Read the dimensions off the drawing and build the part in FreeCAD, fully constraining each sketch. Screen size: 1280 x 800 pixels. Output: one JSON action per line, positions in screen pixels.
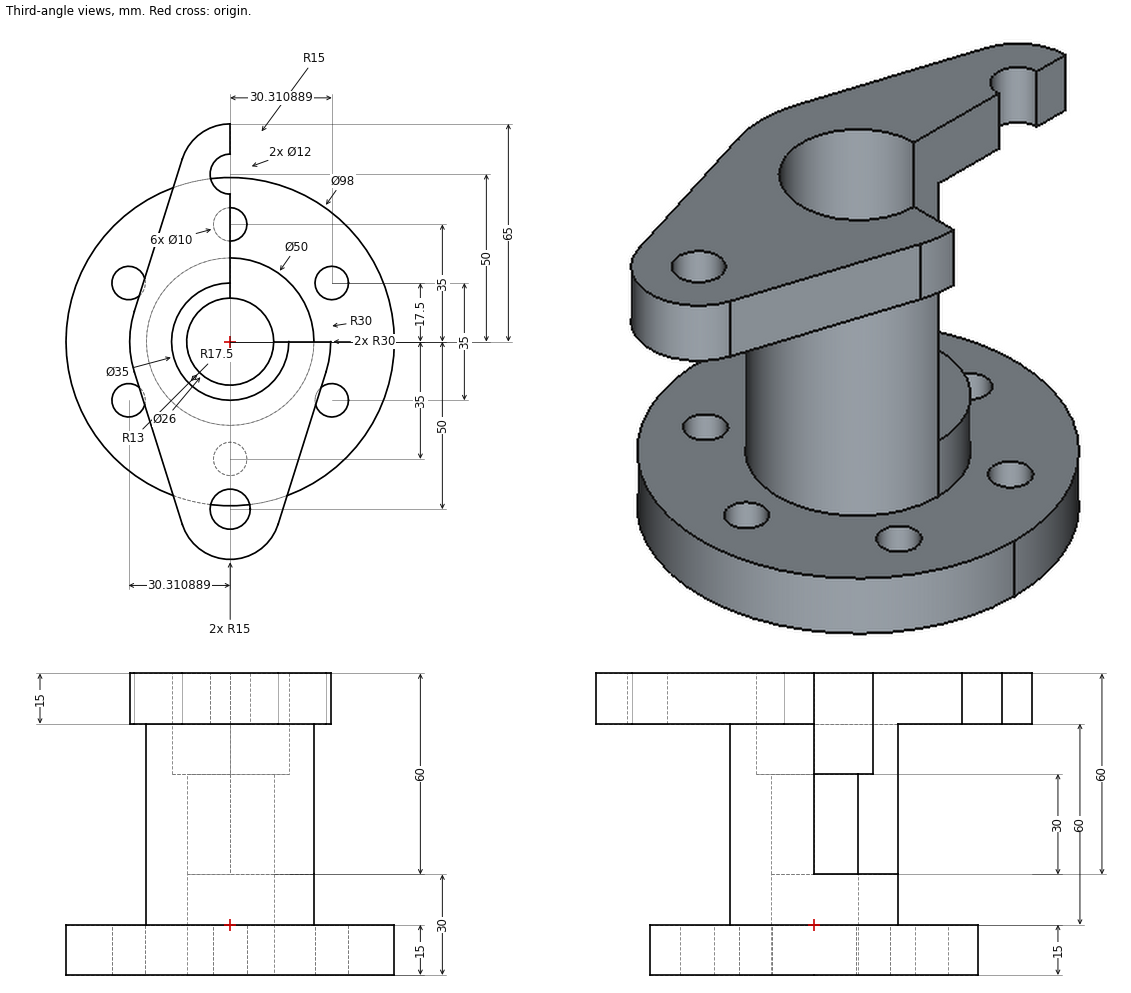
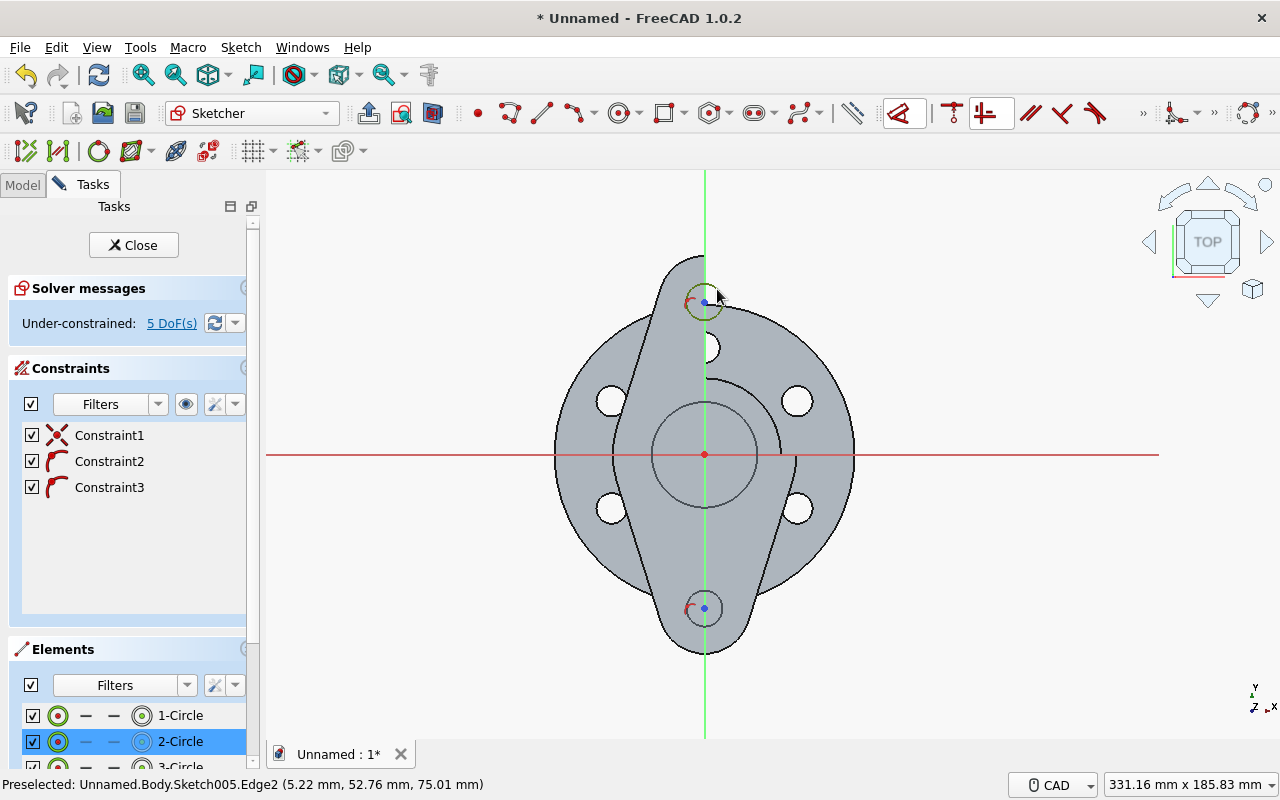
{"action": "left_click", "coordinate": [717, 596]}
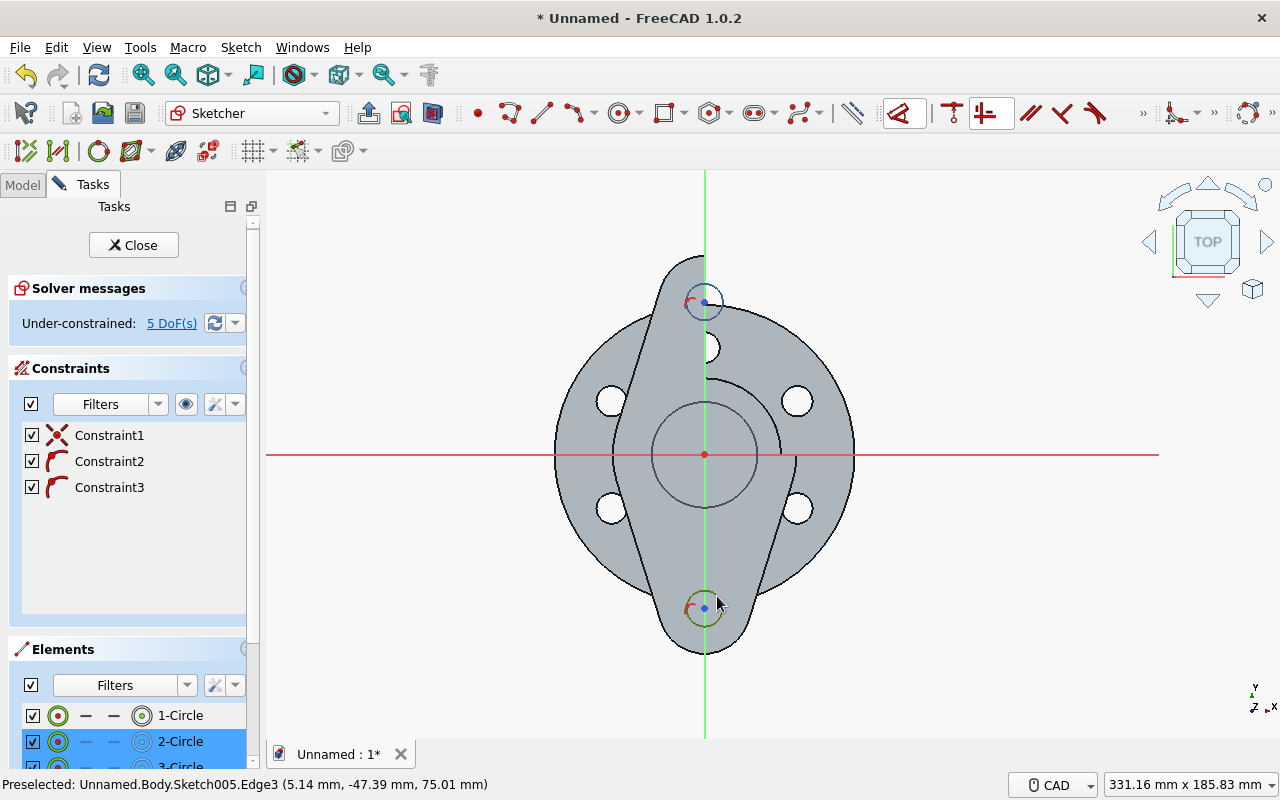
{"action": "key", "text": "e"}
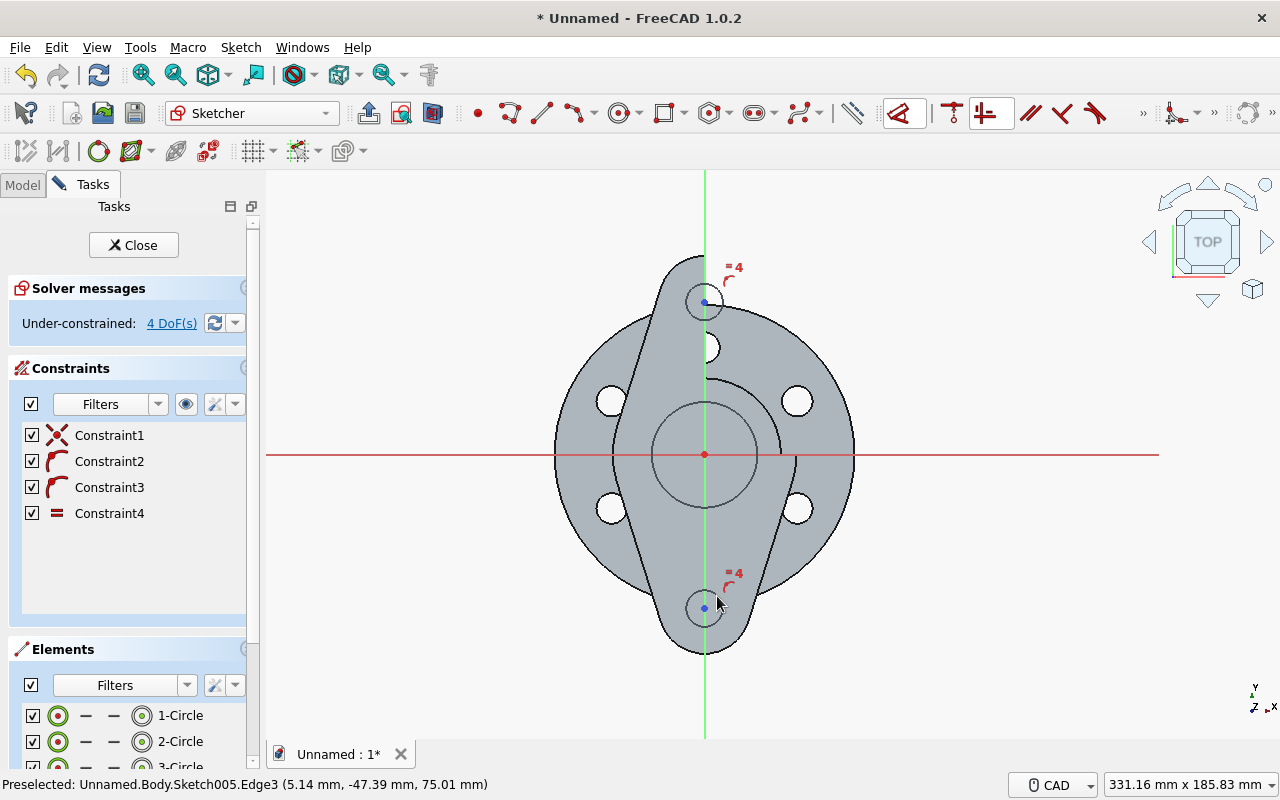
{"action": "left_click", "coordinate": [742, 417]}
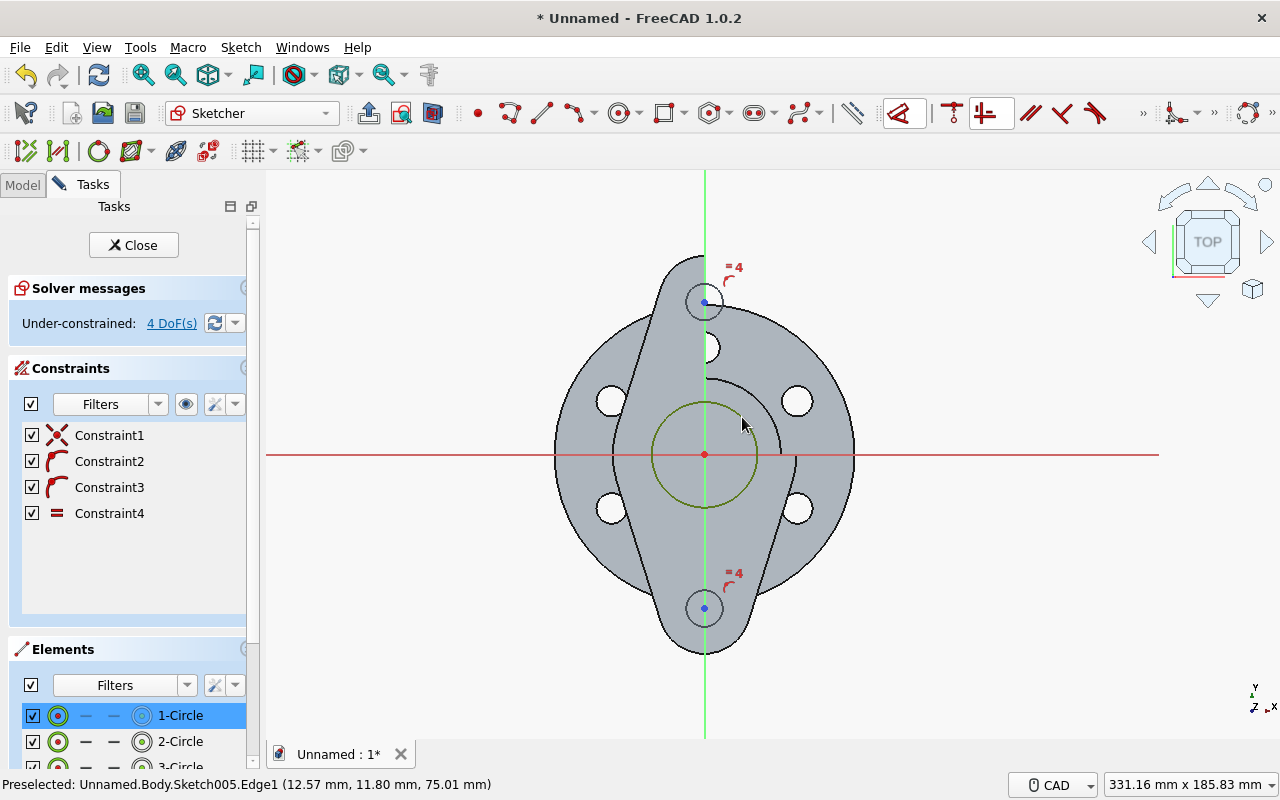
{"action": "key", "text": "k o"}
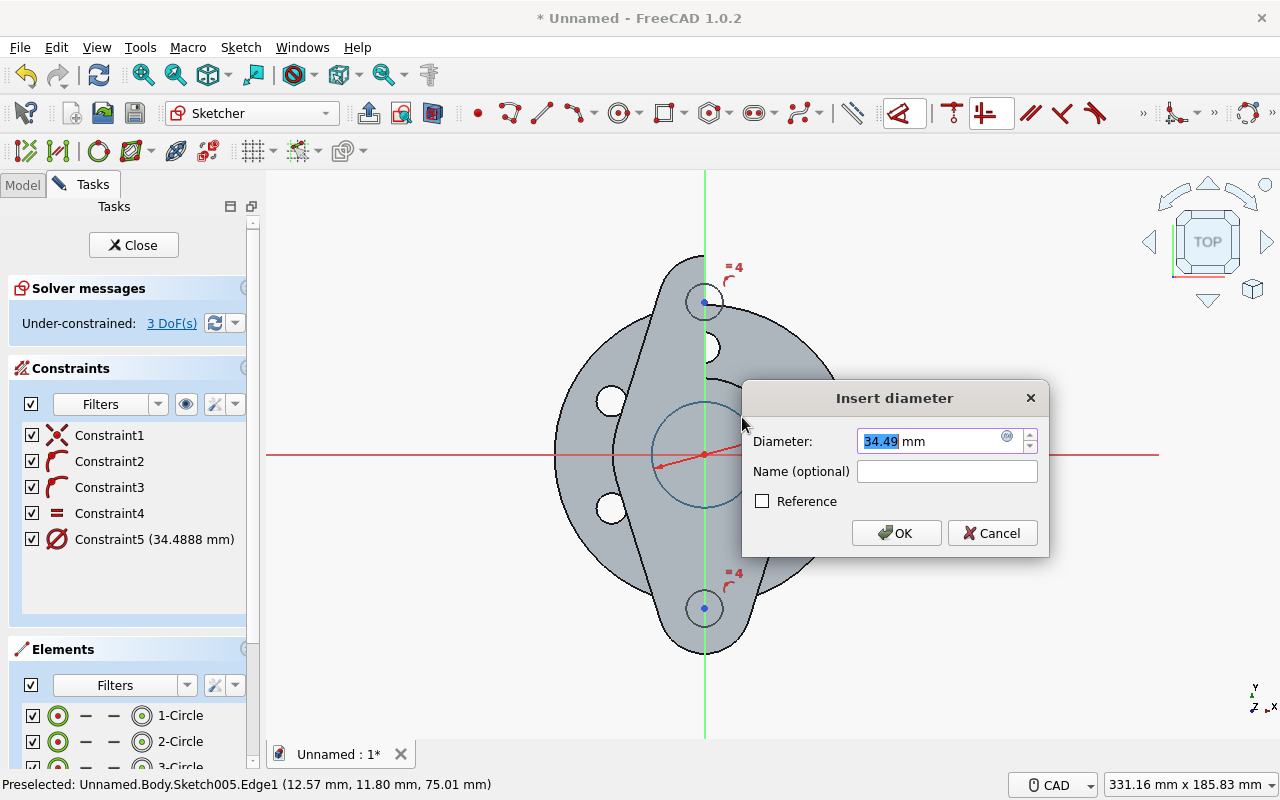
{"action": "type", "text": "35"}
{"action": "key", "text": "Return"}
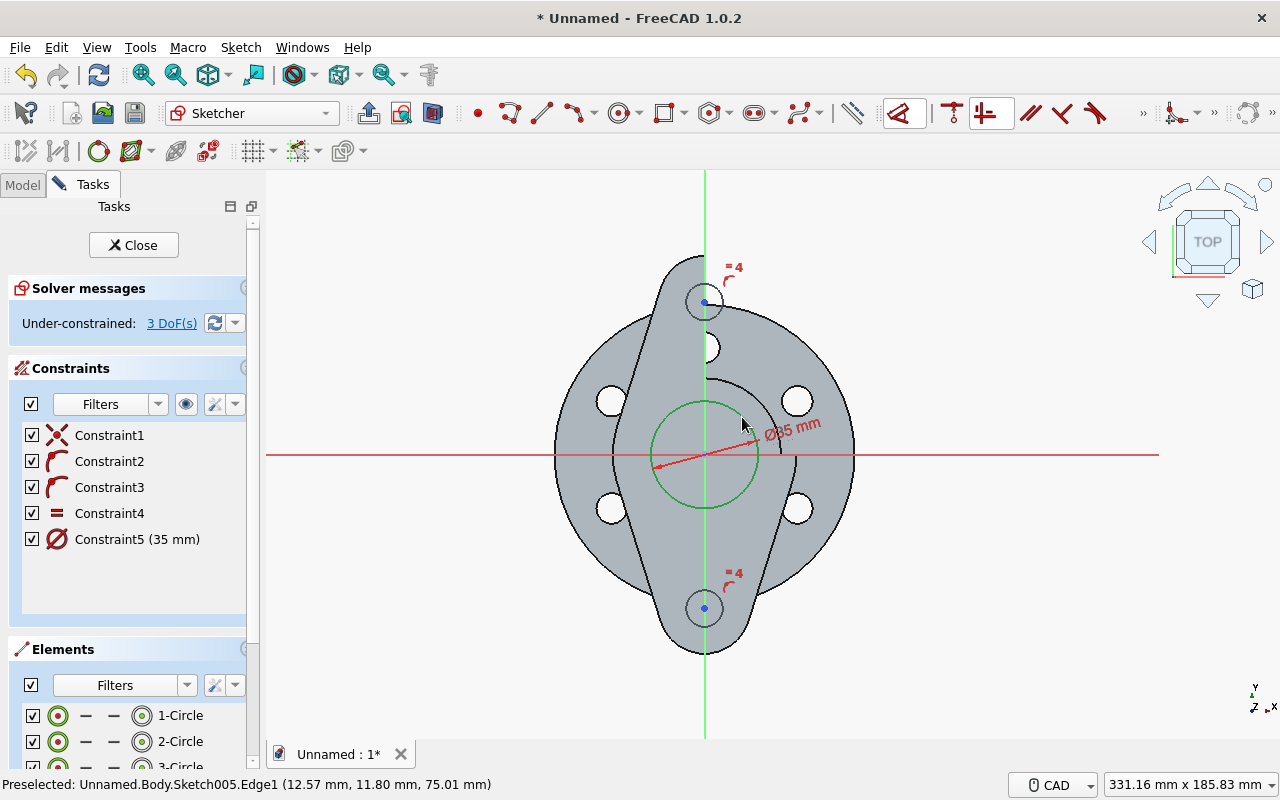
{"action": "left_click", "coordinate": [717, 289]}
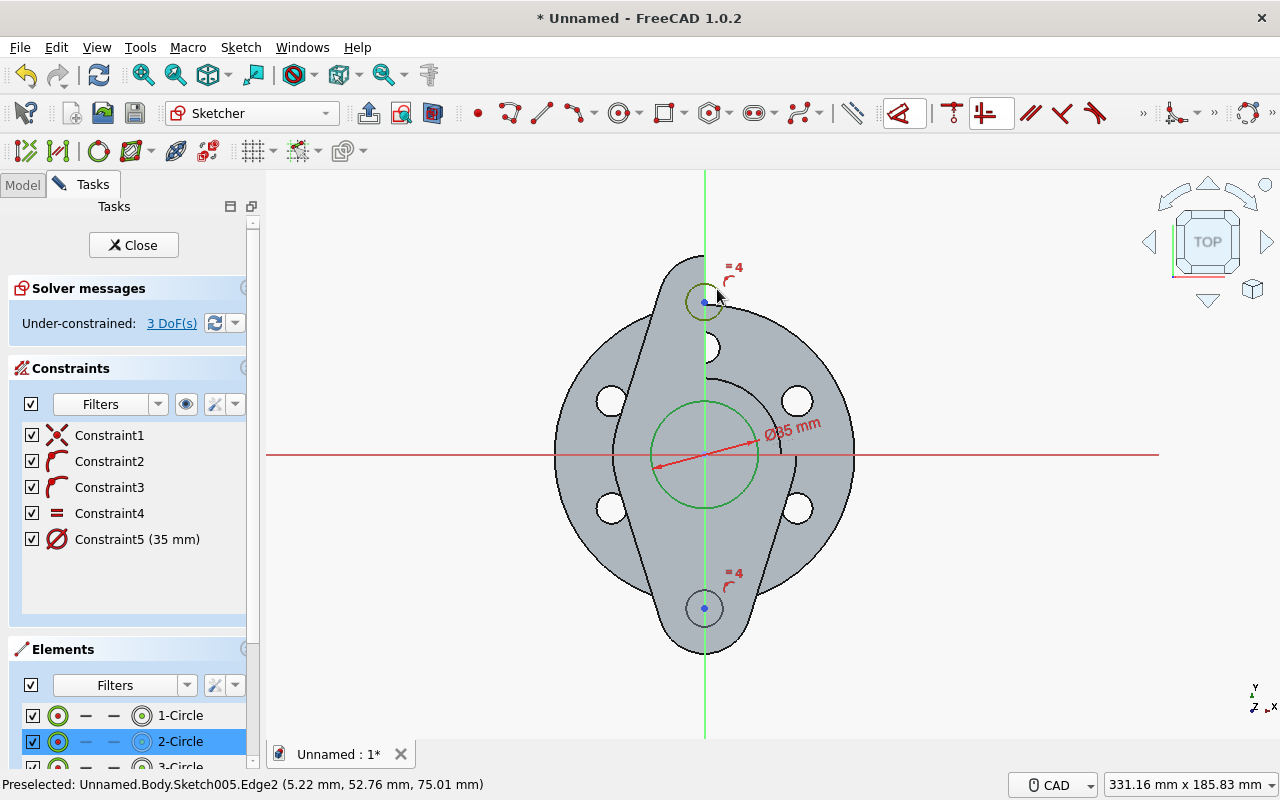
{"action": "key", "text": "k o"}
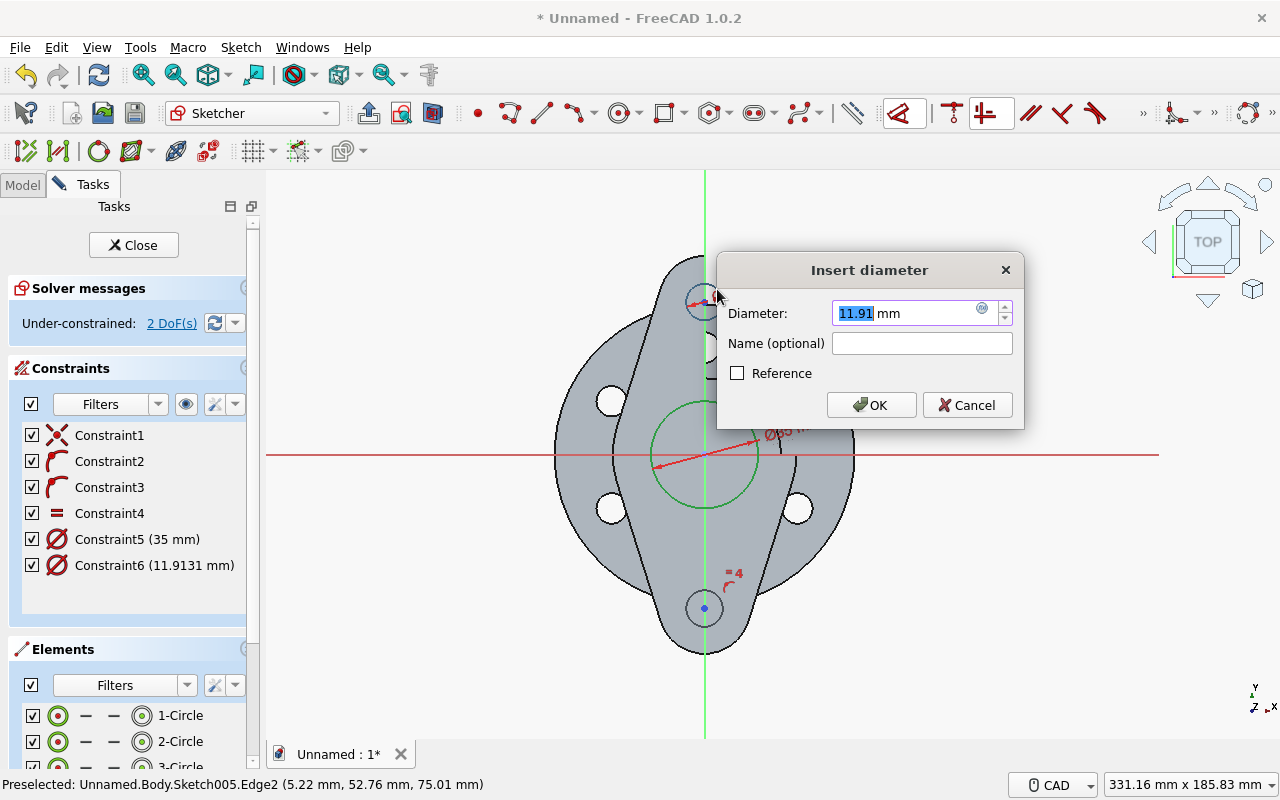
{"action": "type", "text": "12"}
{"action": "key", "text": "Return"}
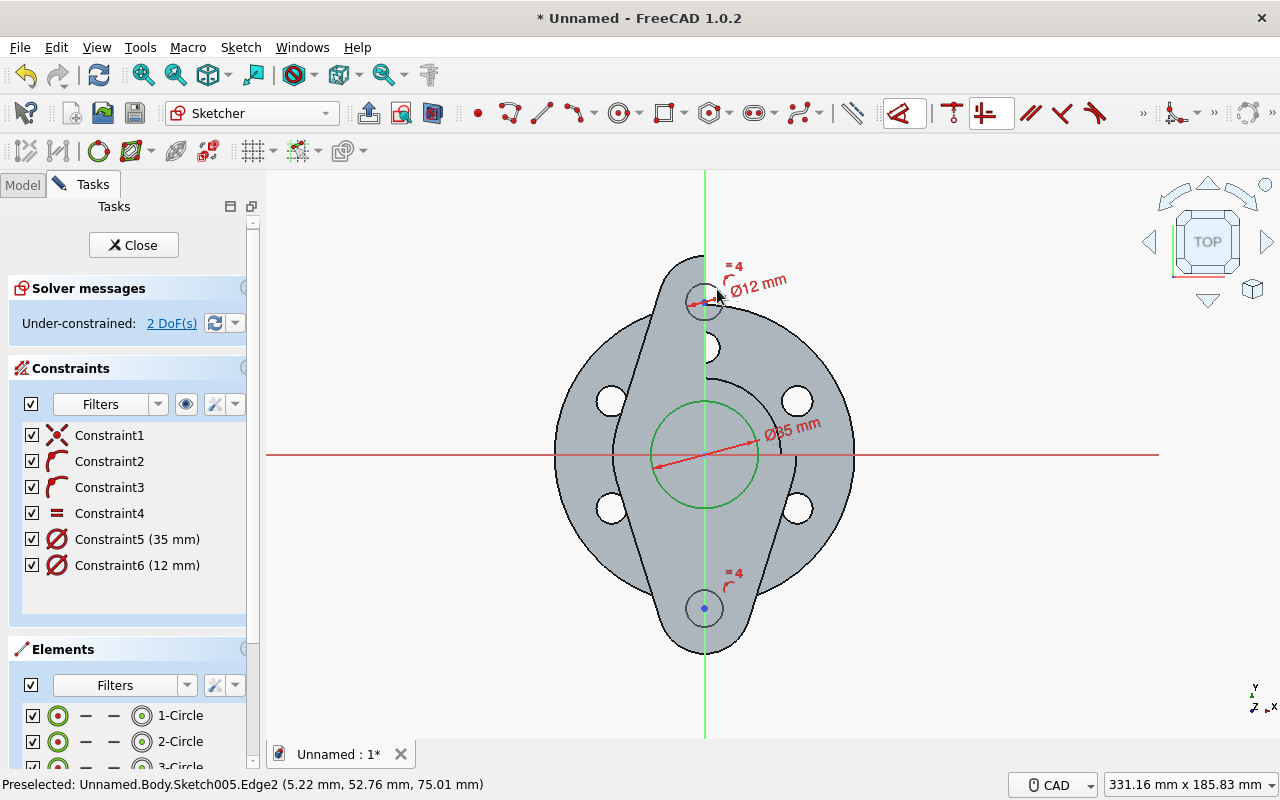
{"action": "left_click", "coordinate": [705, 302]}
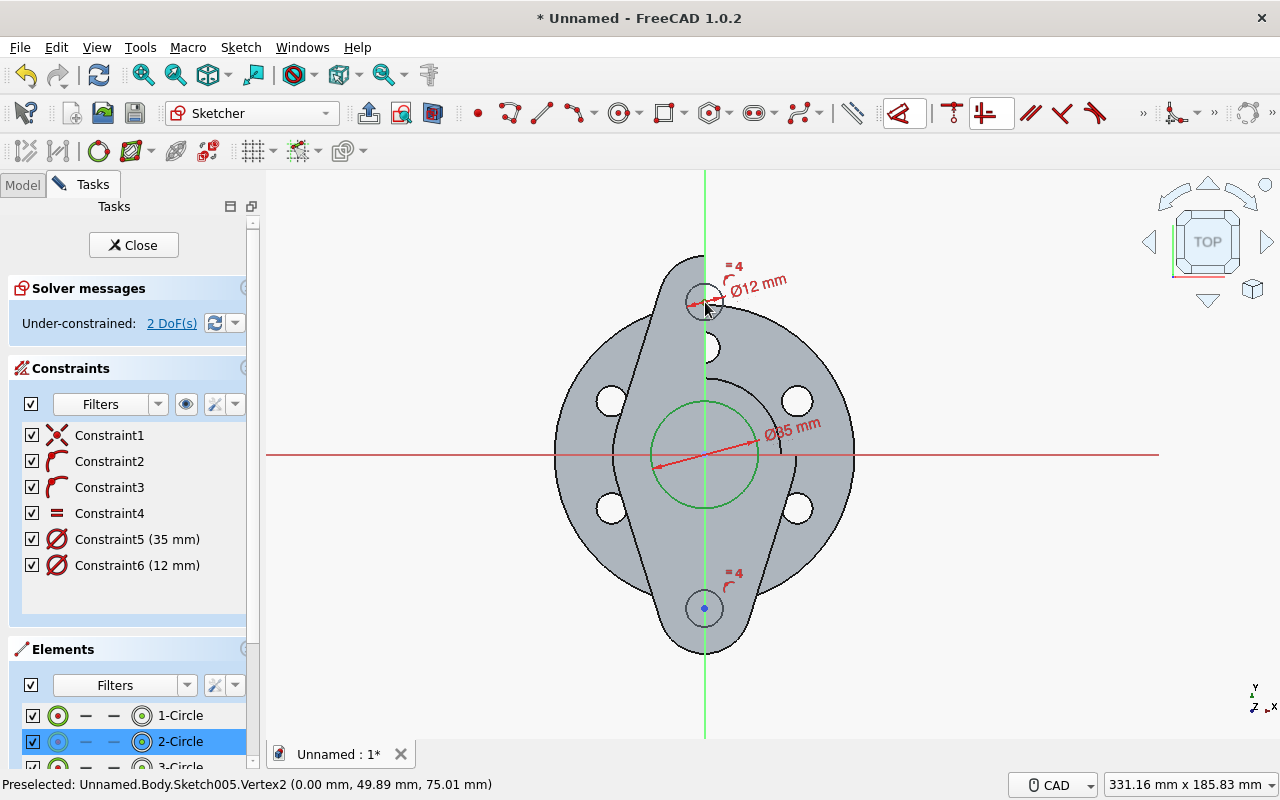
{"action": "key", "text": "i"}